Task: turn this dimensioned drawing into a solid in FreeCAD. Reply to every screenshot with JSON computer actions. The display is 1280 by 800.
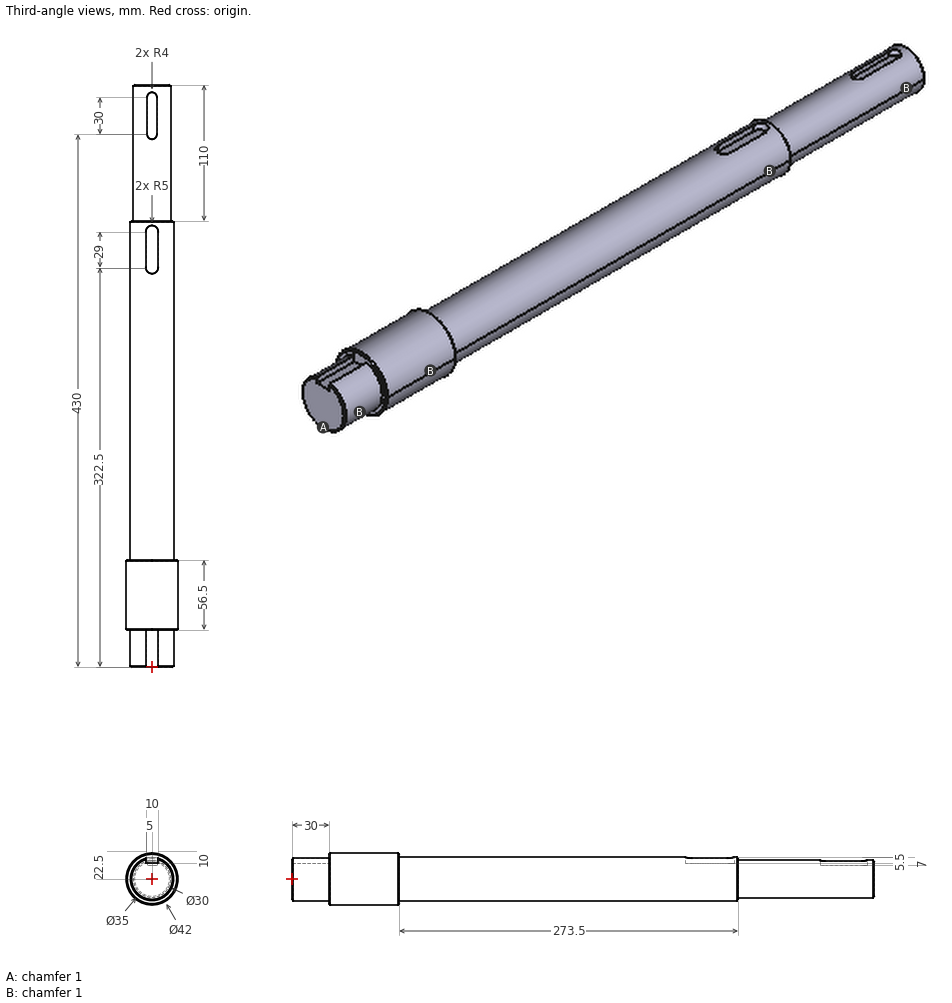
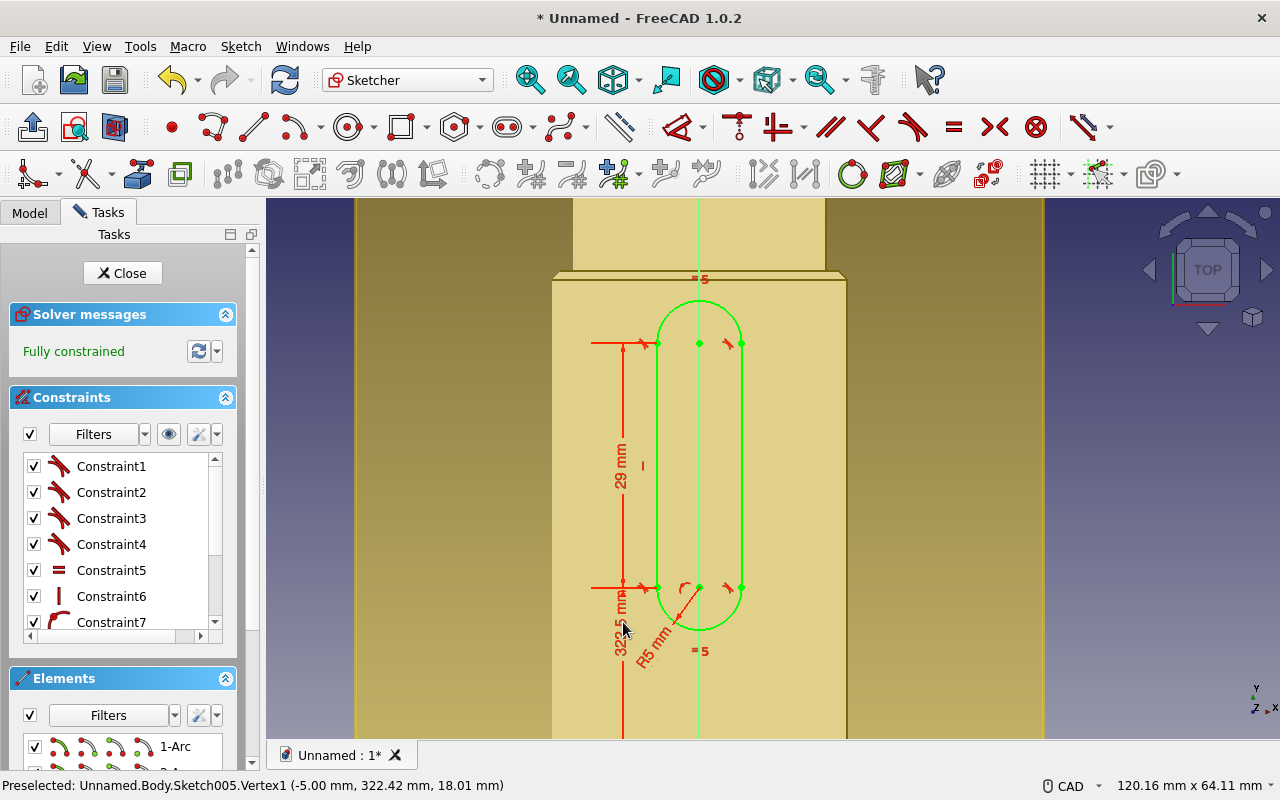
{"action": "left_click", "coordinate": [123, 273]}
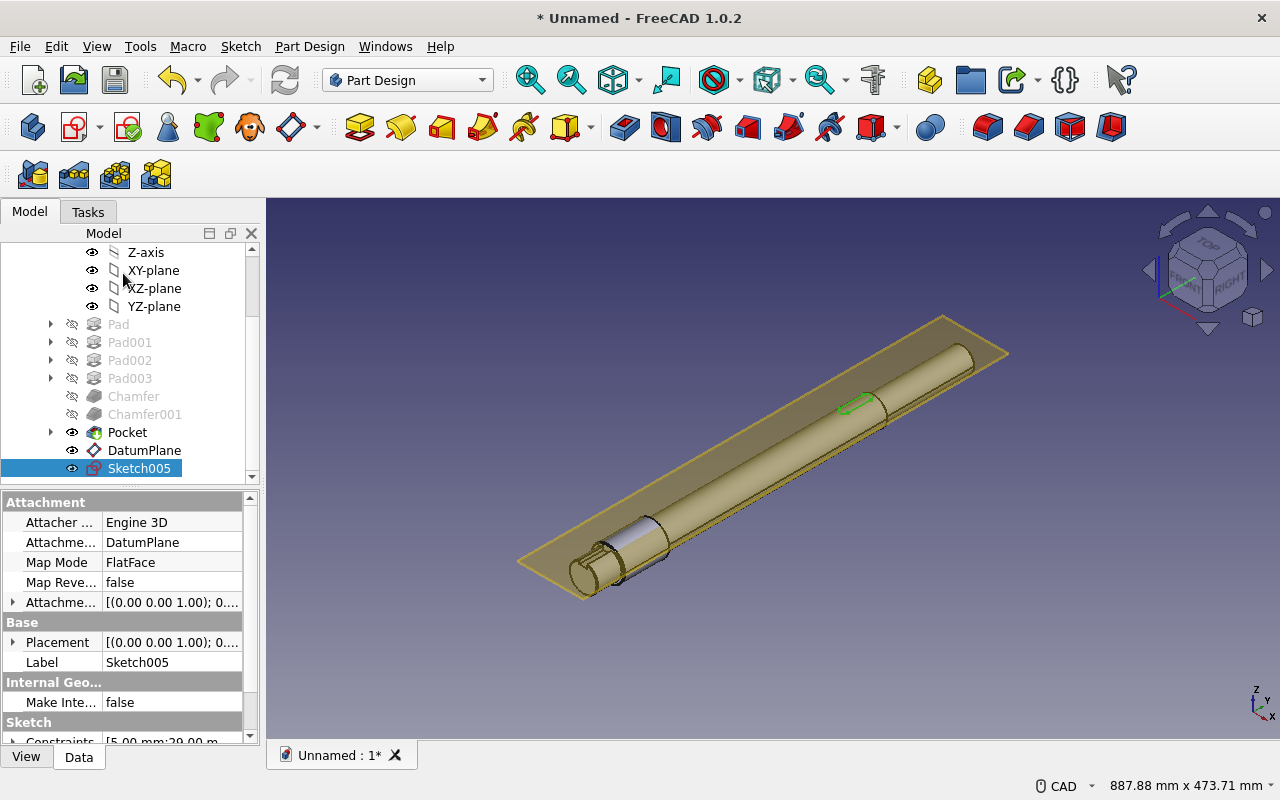
{"action": "left_click", "coordinate": [625, 128]}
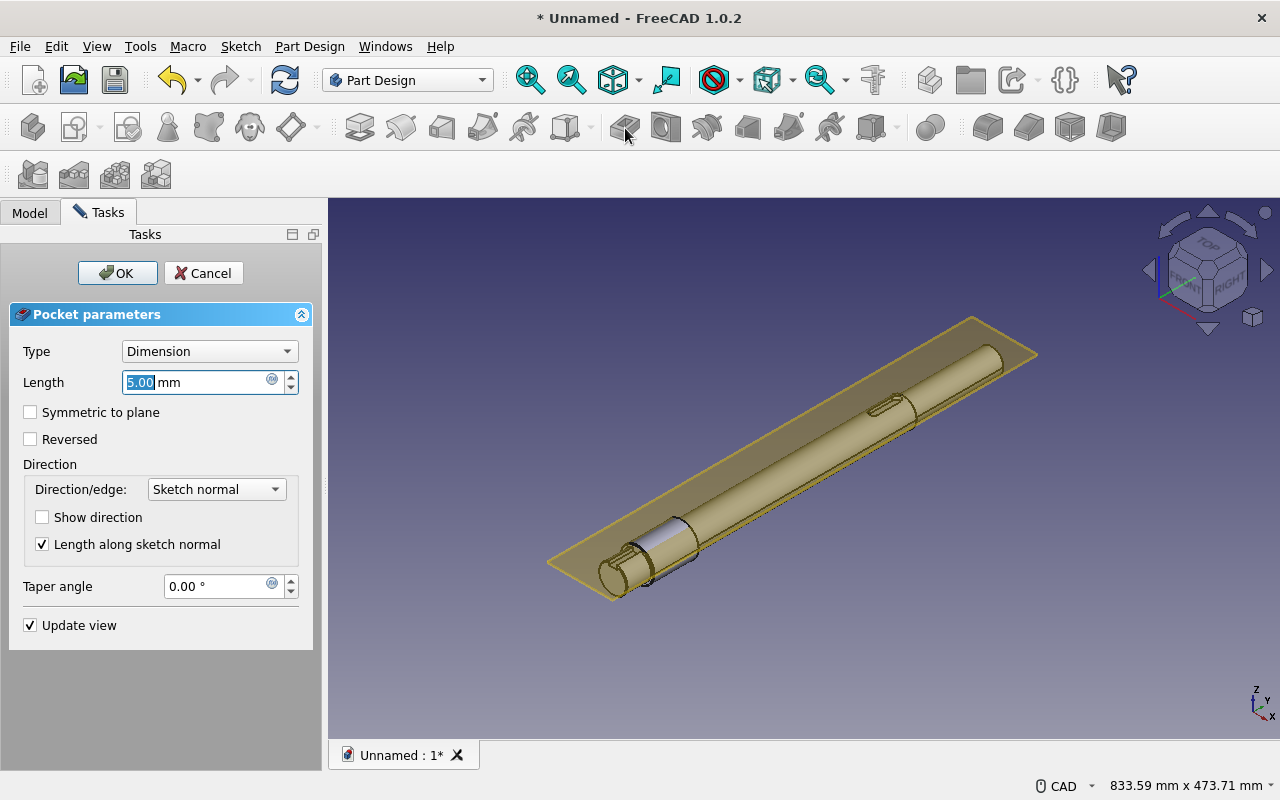
{"action": "type", "text": "5.5"}
{"action": "key", "text": "Tab"}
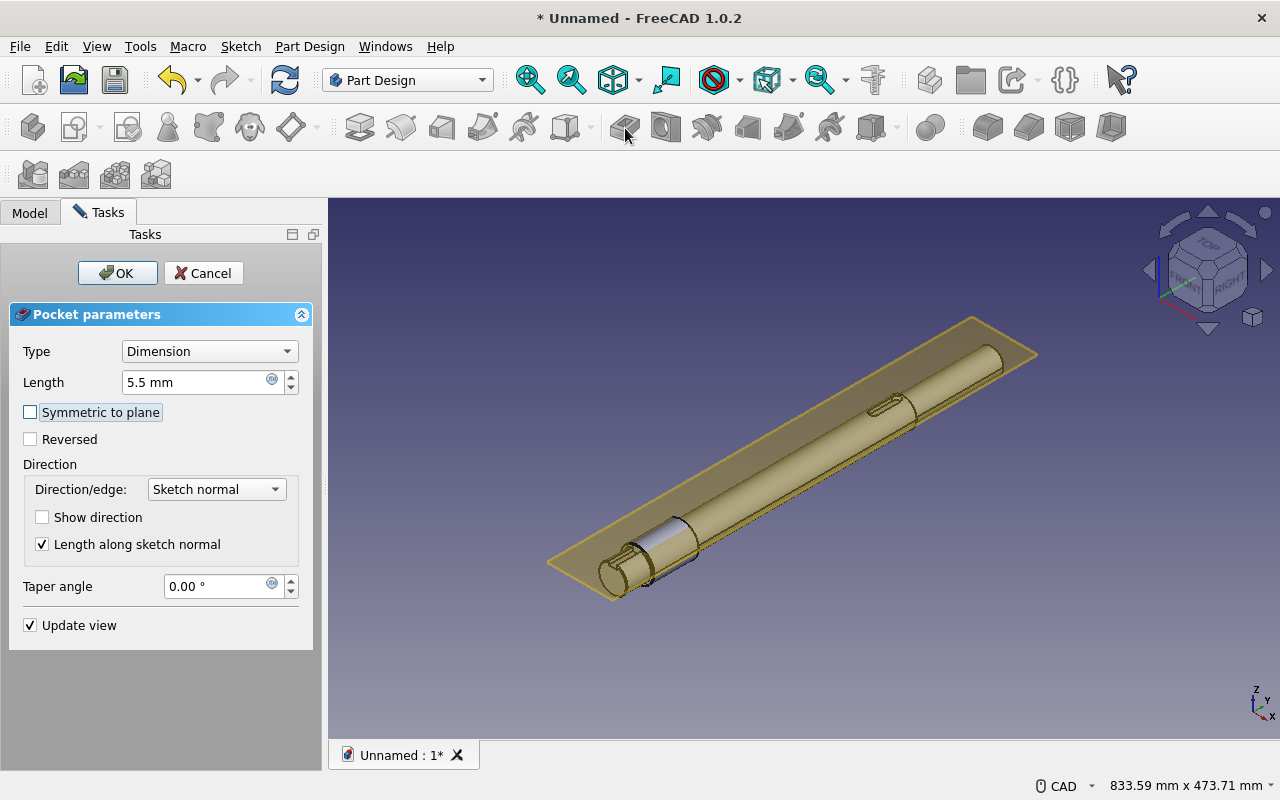
{"action": "left_click", "coordinate": [118, 273]}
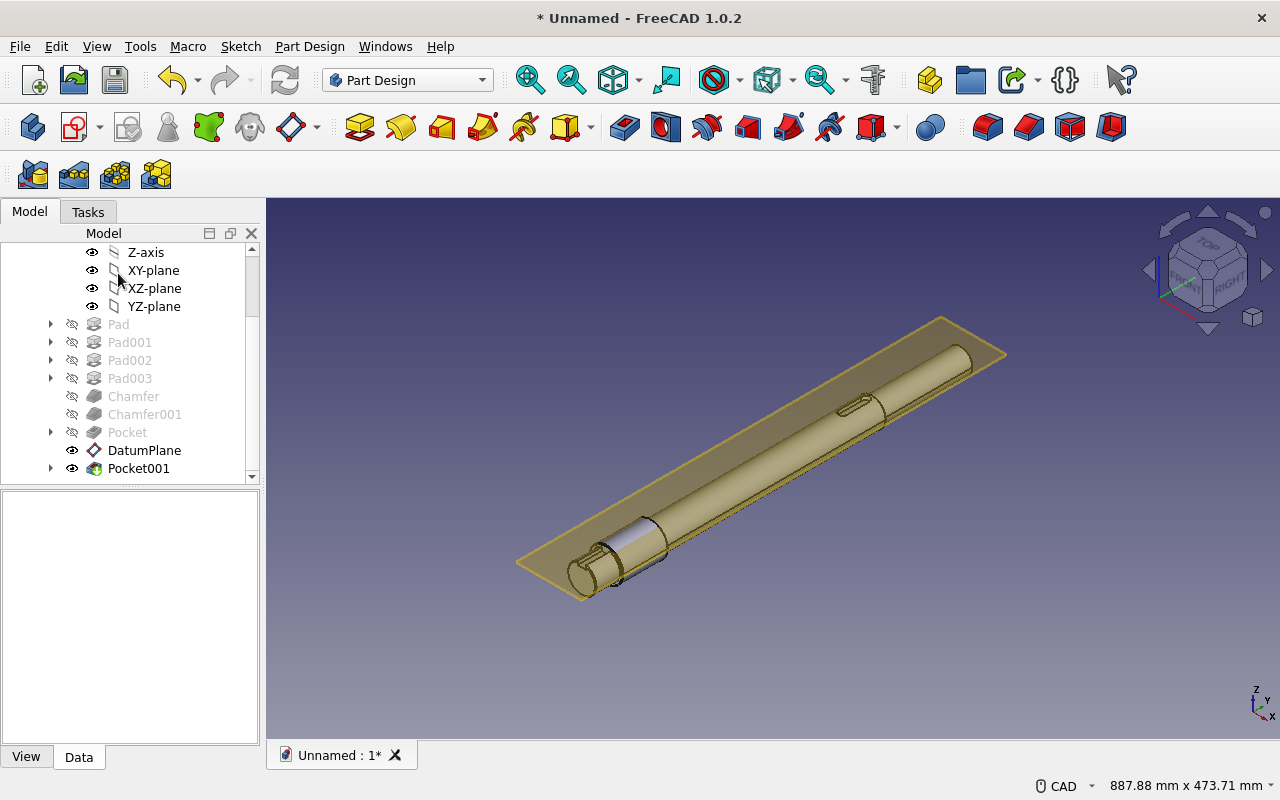
{"action": "left_click", "coordinate": [117, 450]}
{"action": "key", "text": "space"}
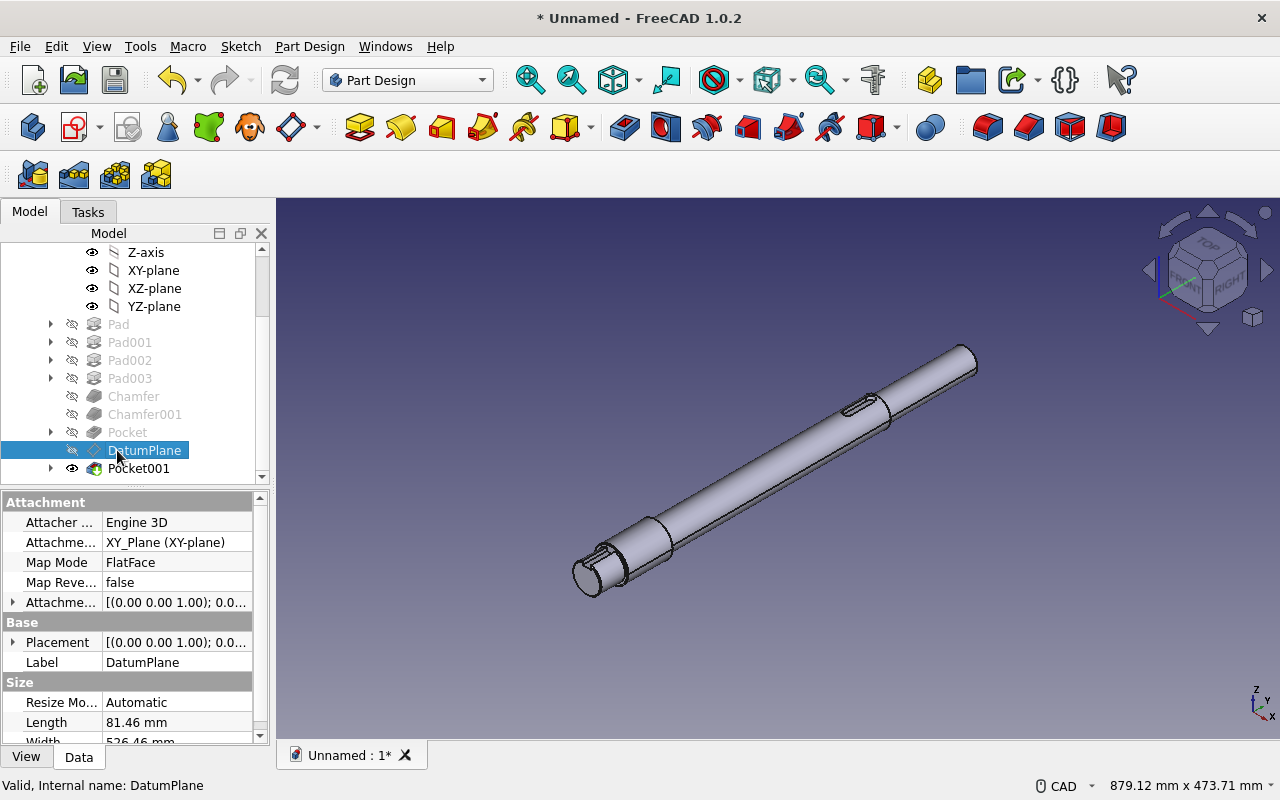
{"action": "scroll", "coordinate": [161, 356], "scroll_direction": "down", "scroll_amount": 3}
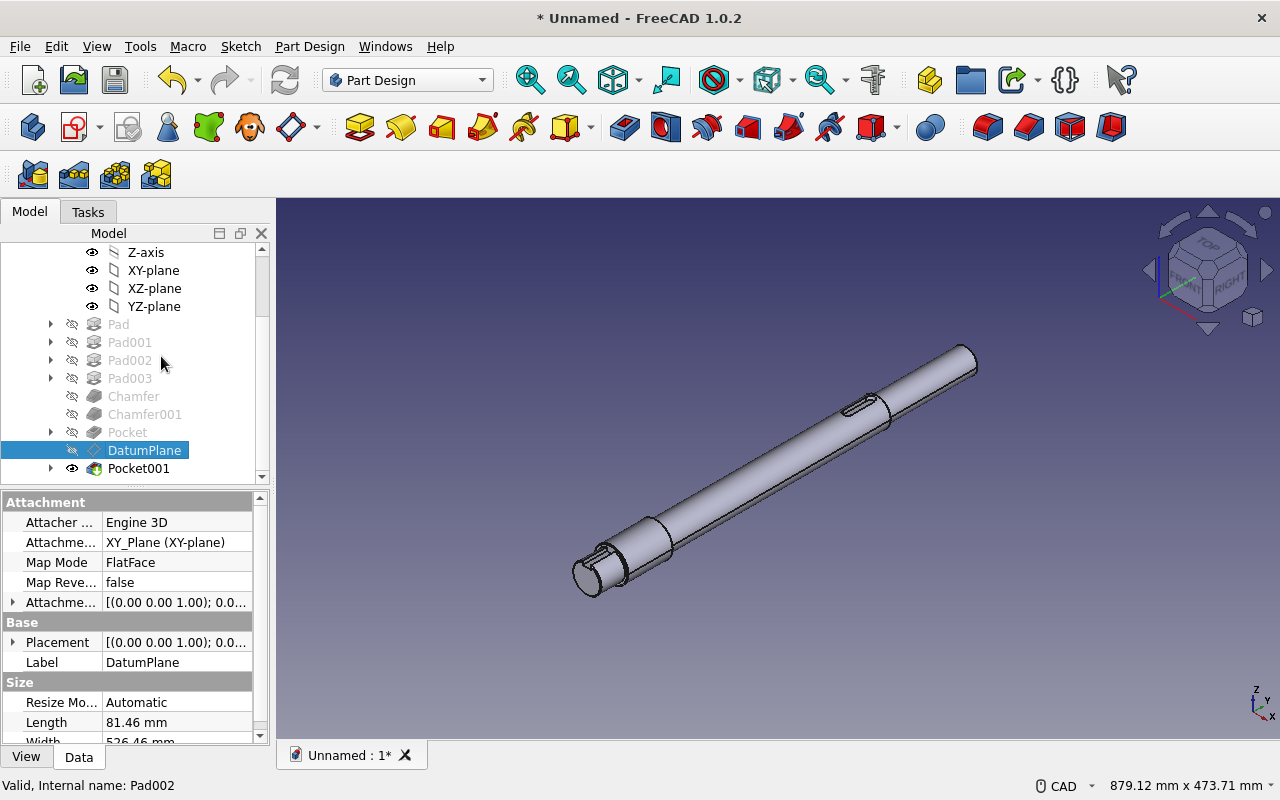
{"action": "scroll", "coordinate": [161, 356], "scroll_direction": "up", "scroll_amount": 15}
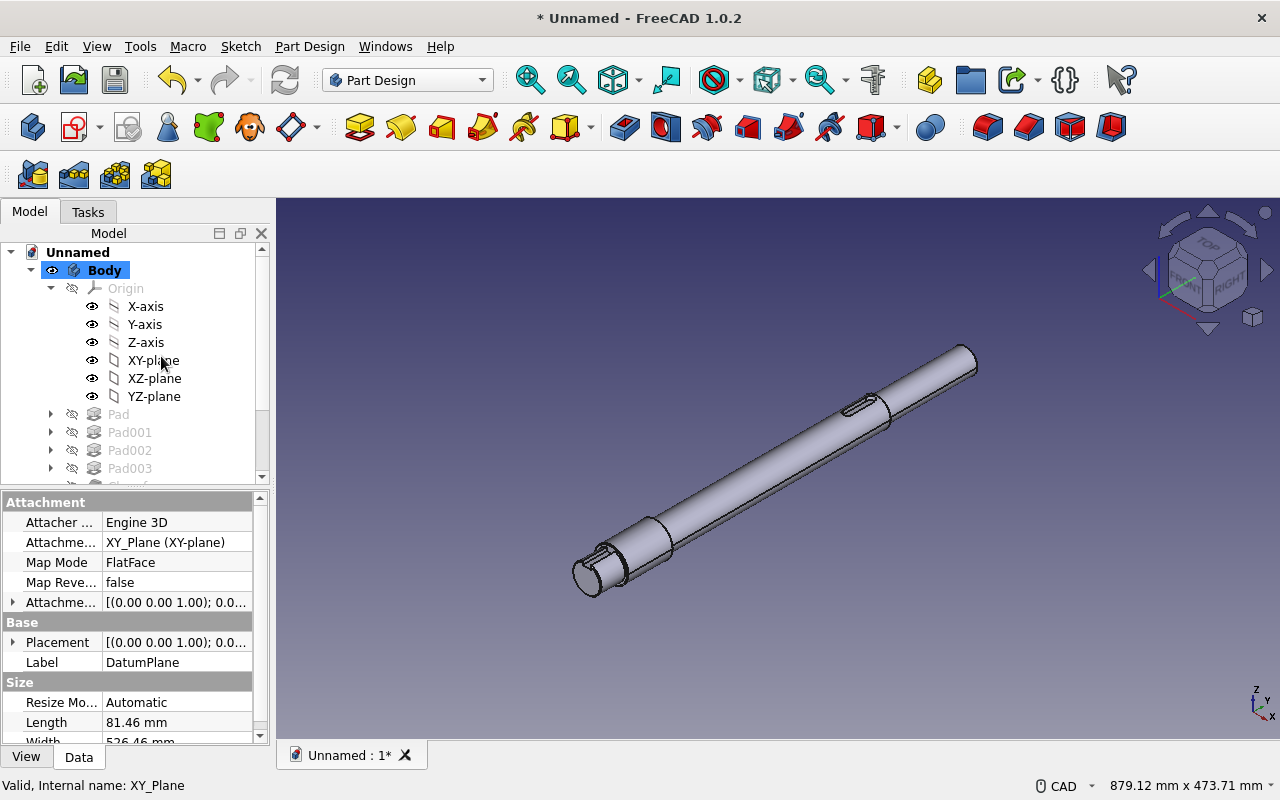
{"action": "left_click", "coordinate": [137, 360]}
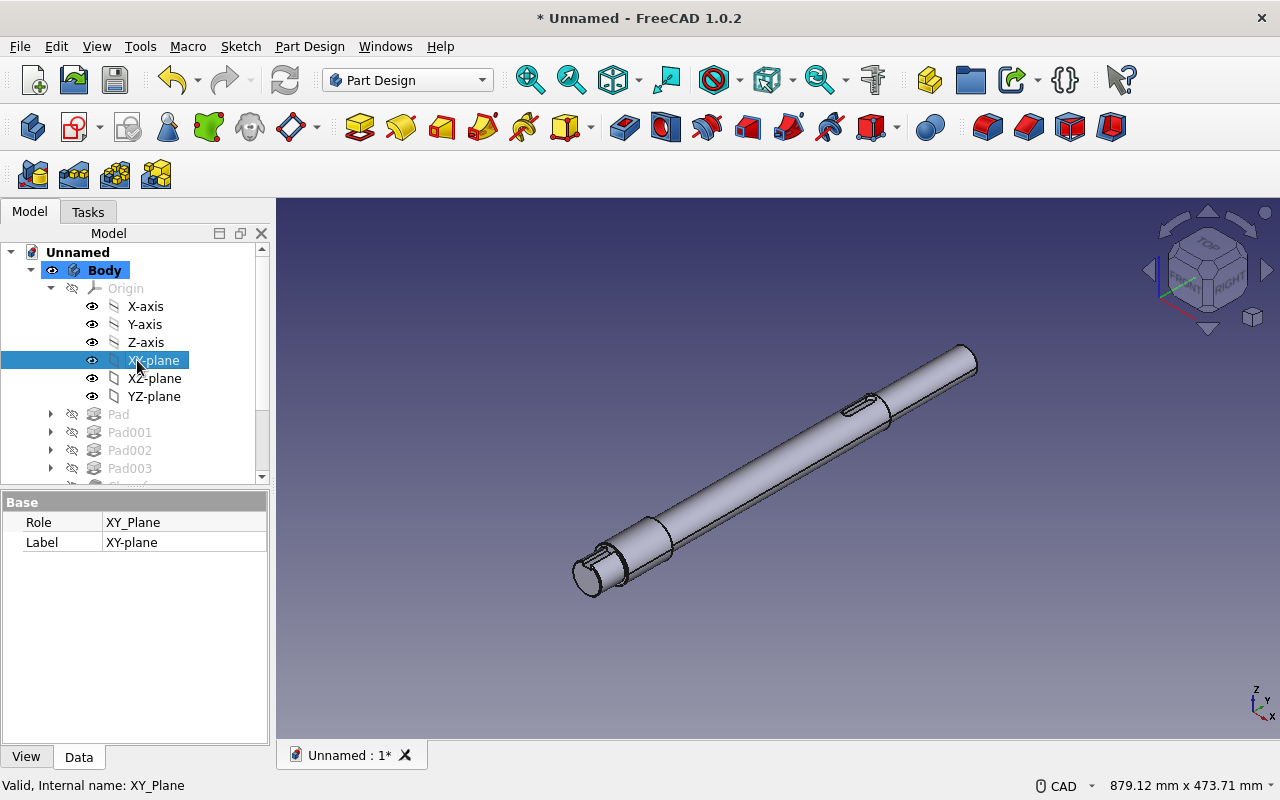
{"action": "left_click", "coordinate": [290, 128]}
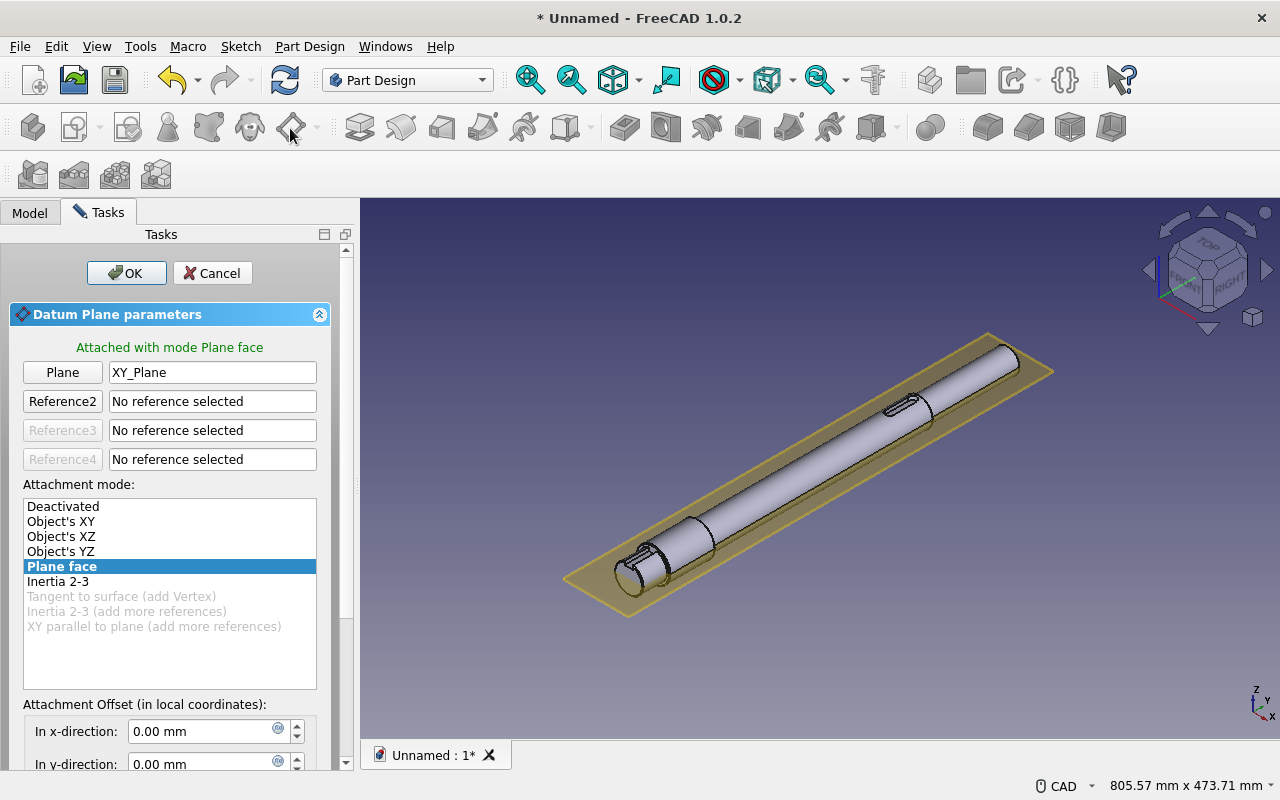
{"action": "scroll", "coordinate": [346, 507], "scroll_direction": "down", "scroll_amount": 2}